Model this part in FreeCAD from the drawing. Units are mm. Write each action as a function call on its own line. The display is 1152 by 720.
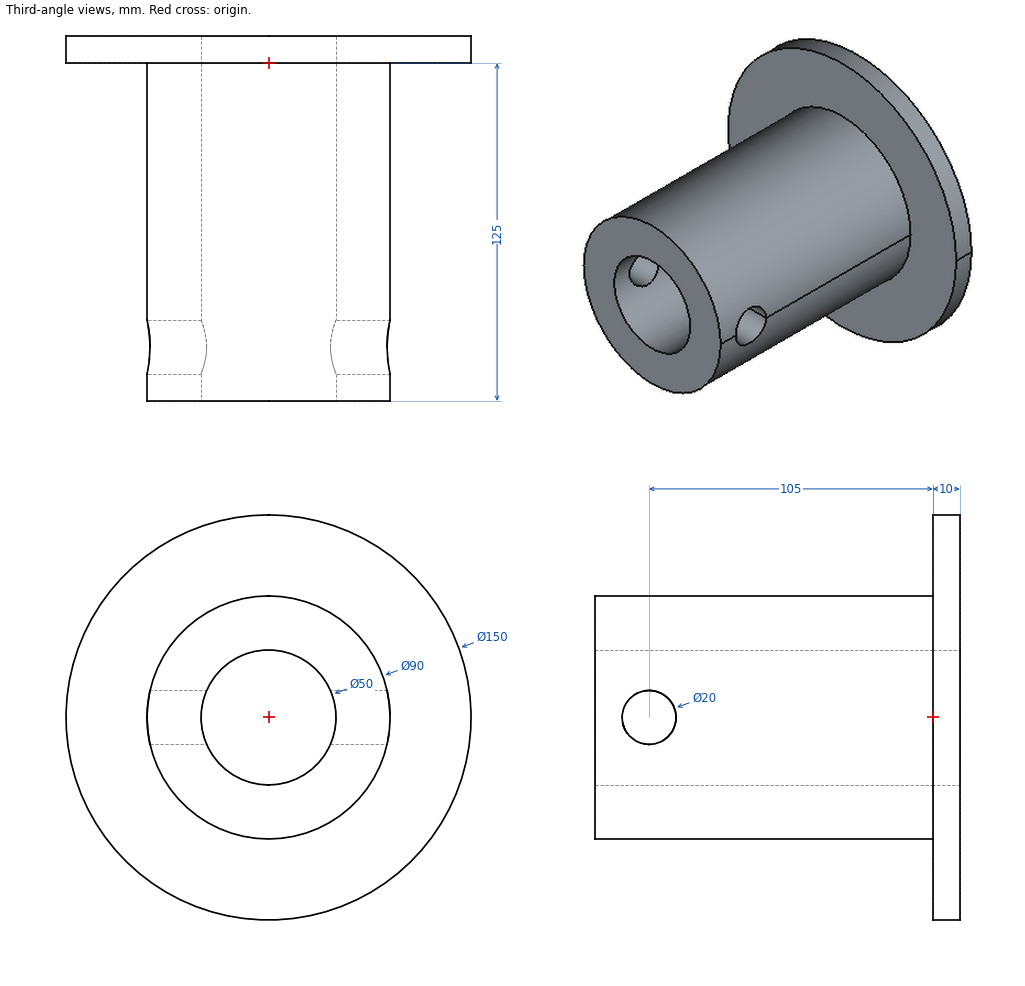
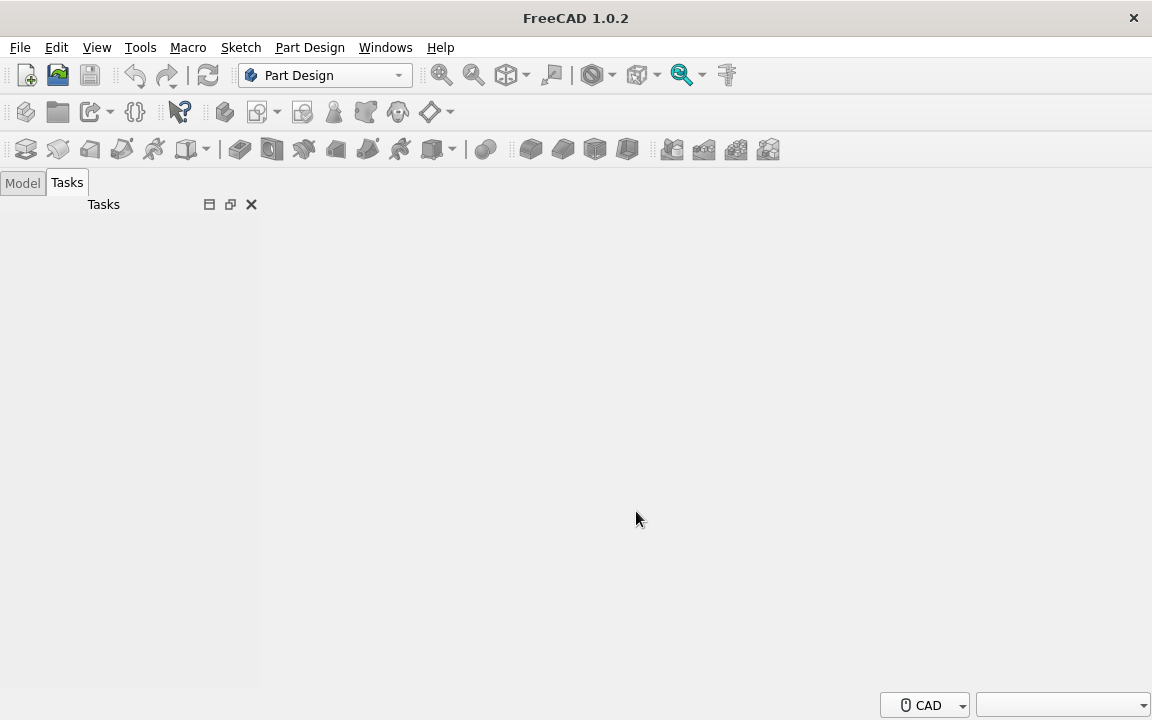
click(26, 76)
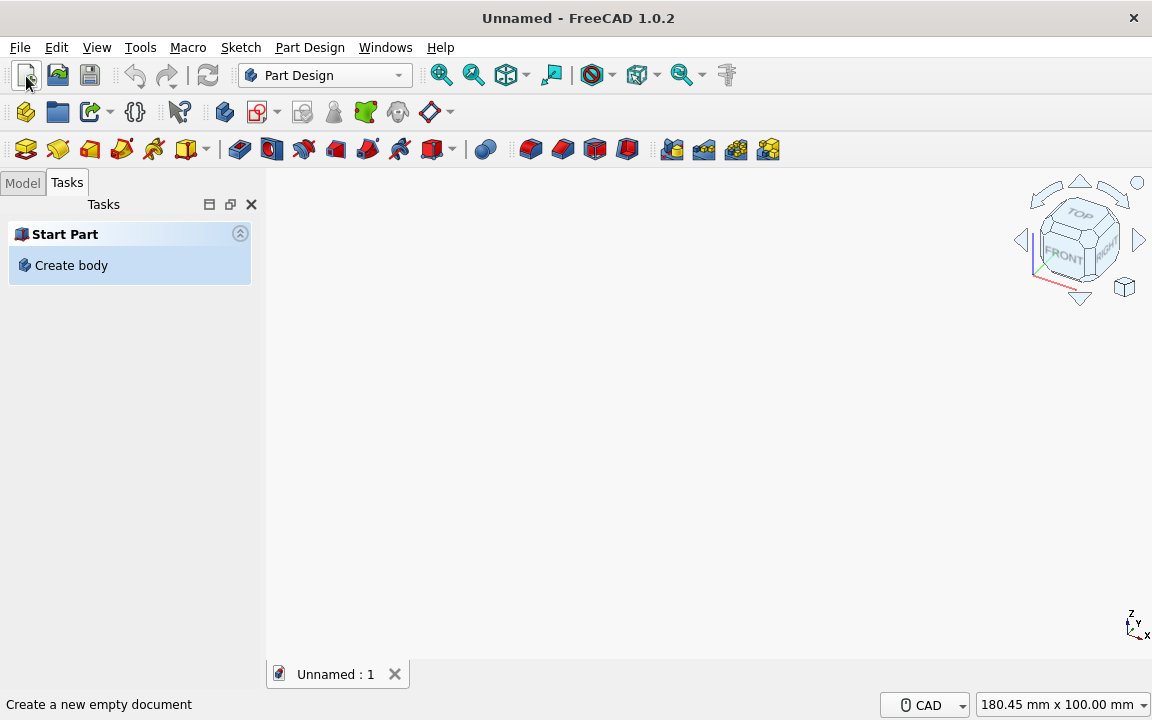
click(258, 112)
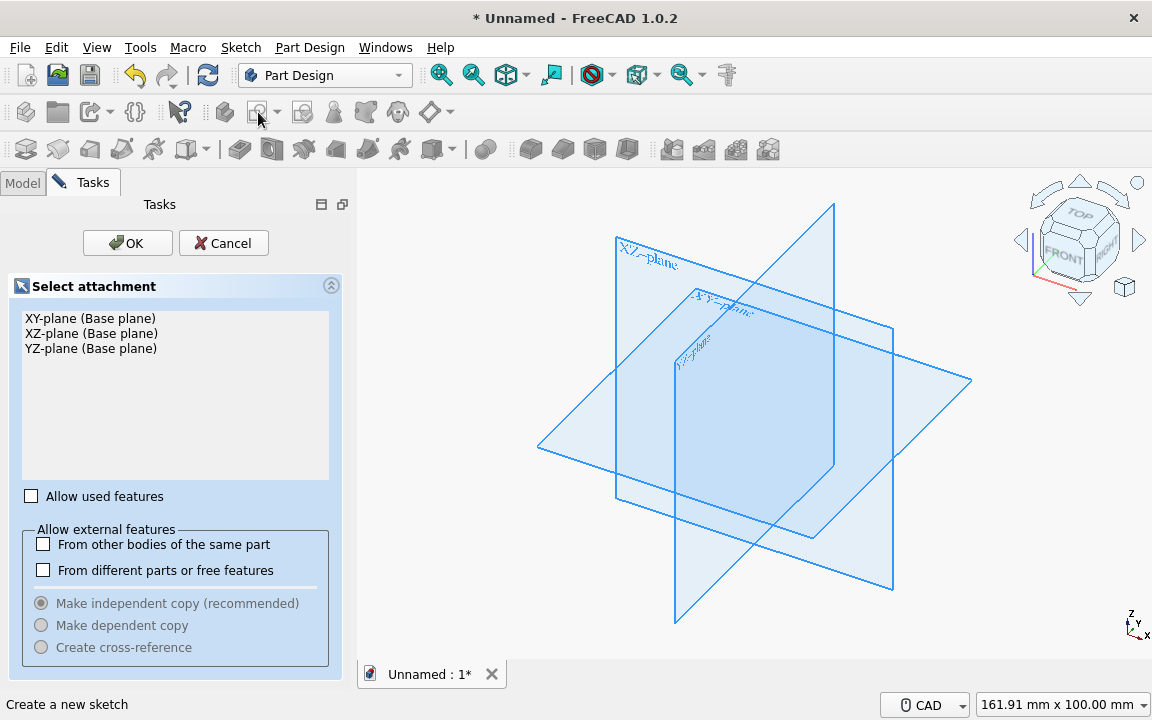
click(82, 334)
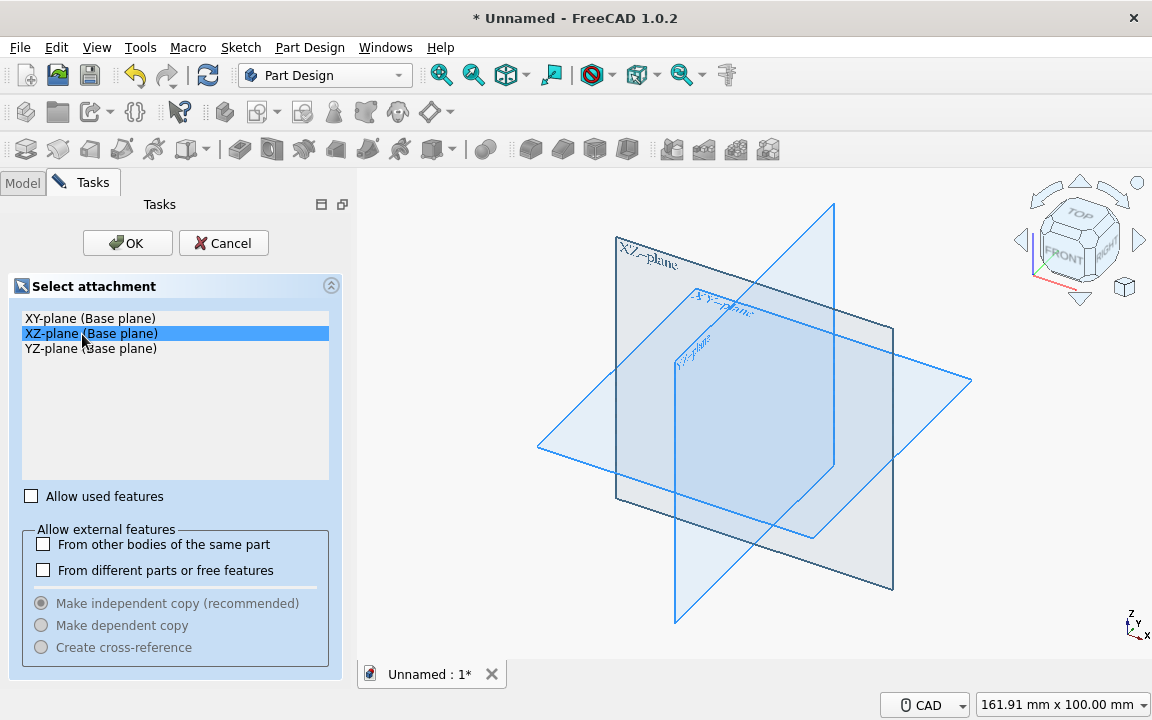
click(128, 243)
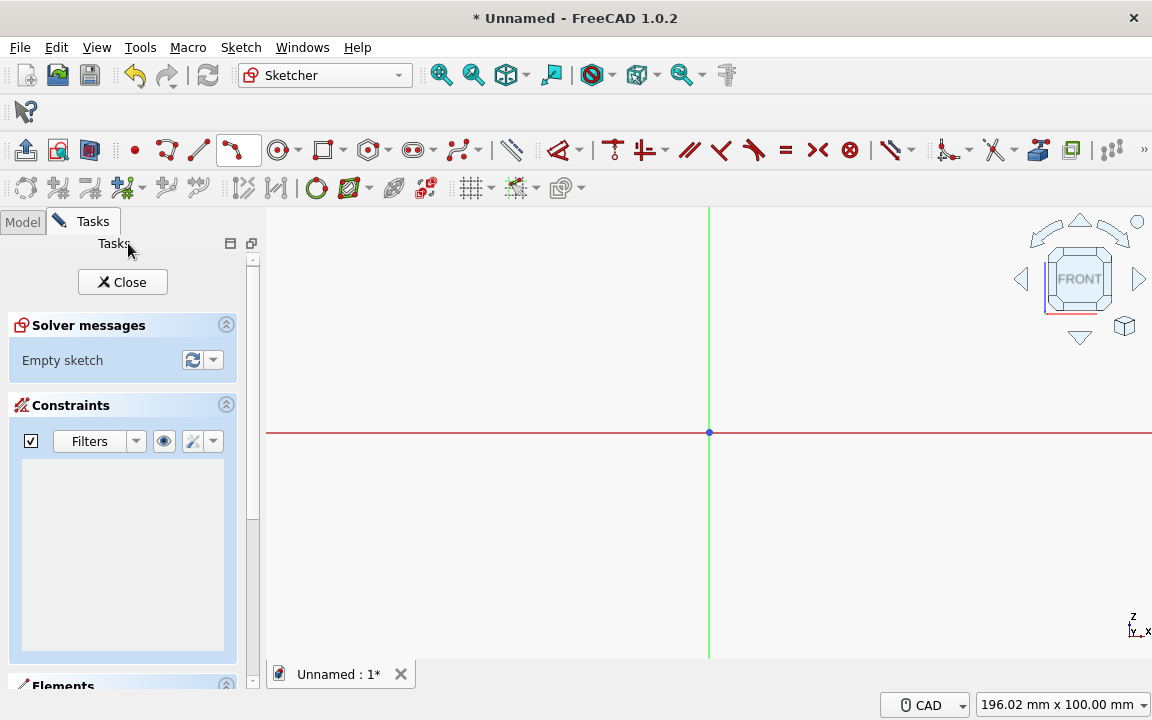
scroll(585, 433, down, 4)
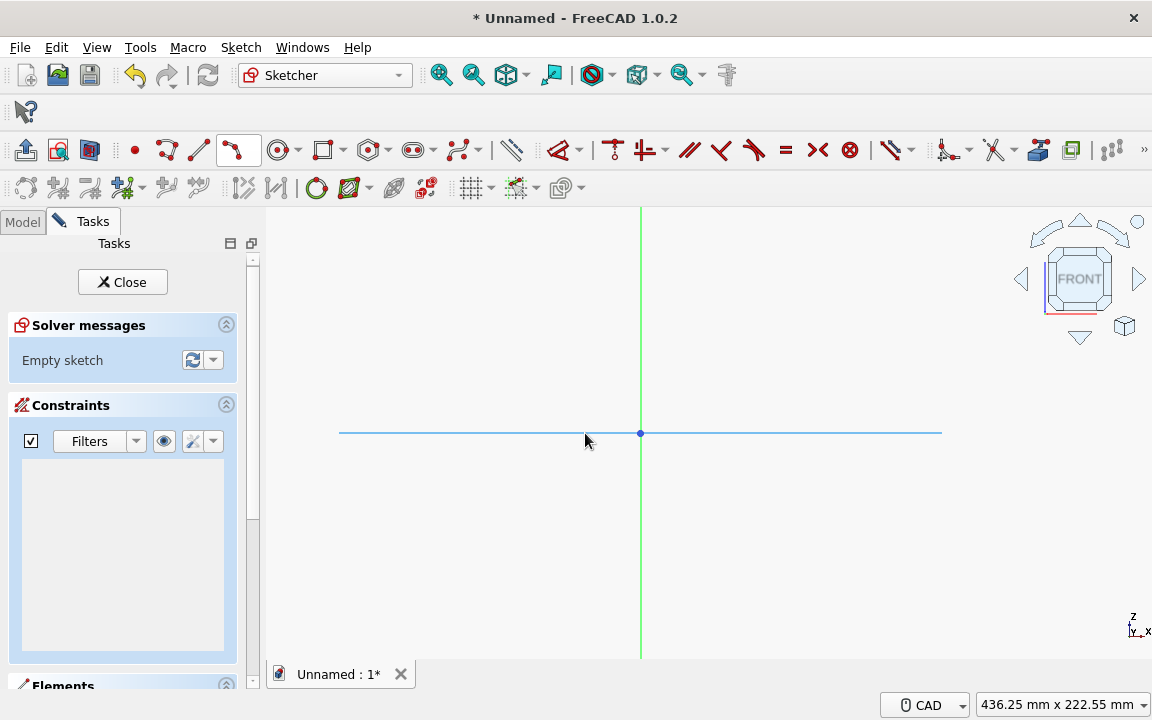
click(278, 150)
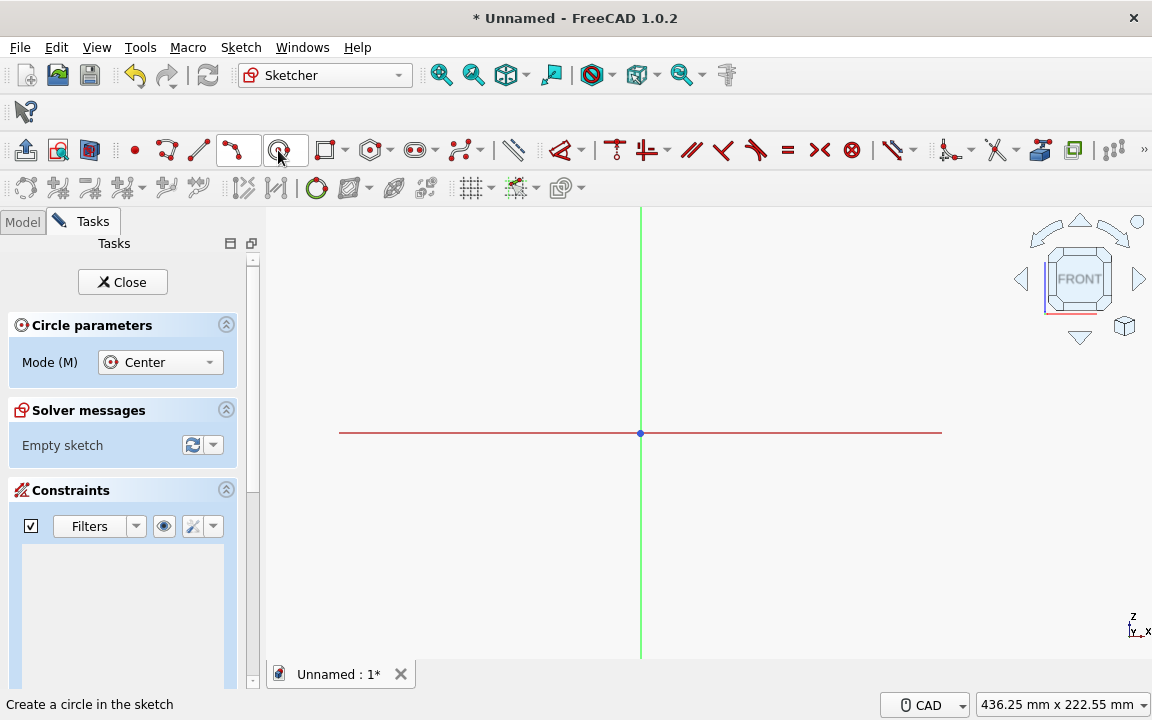
click(641, 433)
click(749, 326)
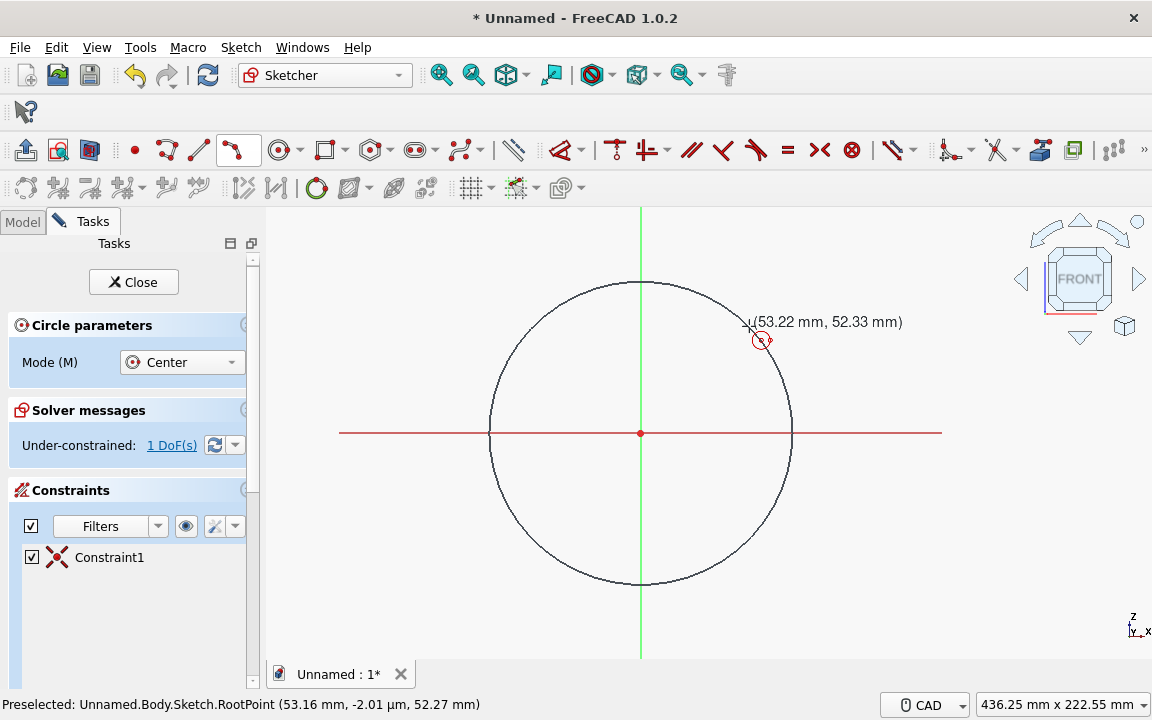
click(641, 433)
click(677, 397)
key(Escape)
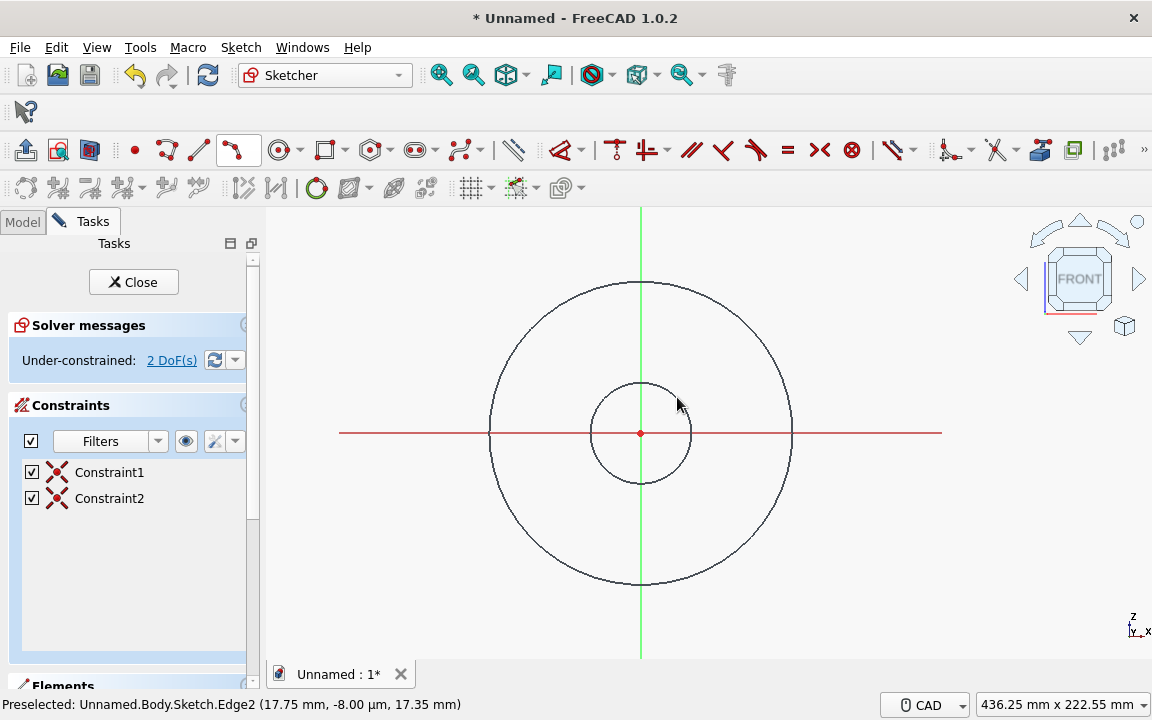
click(560, 150)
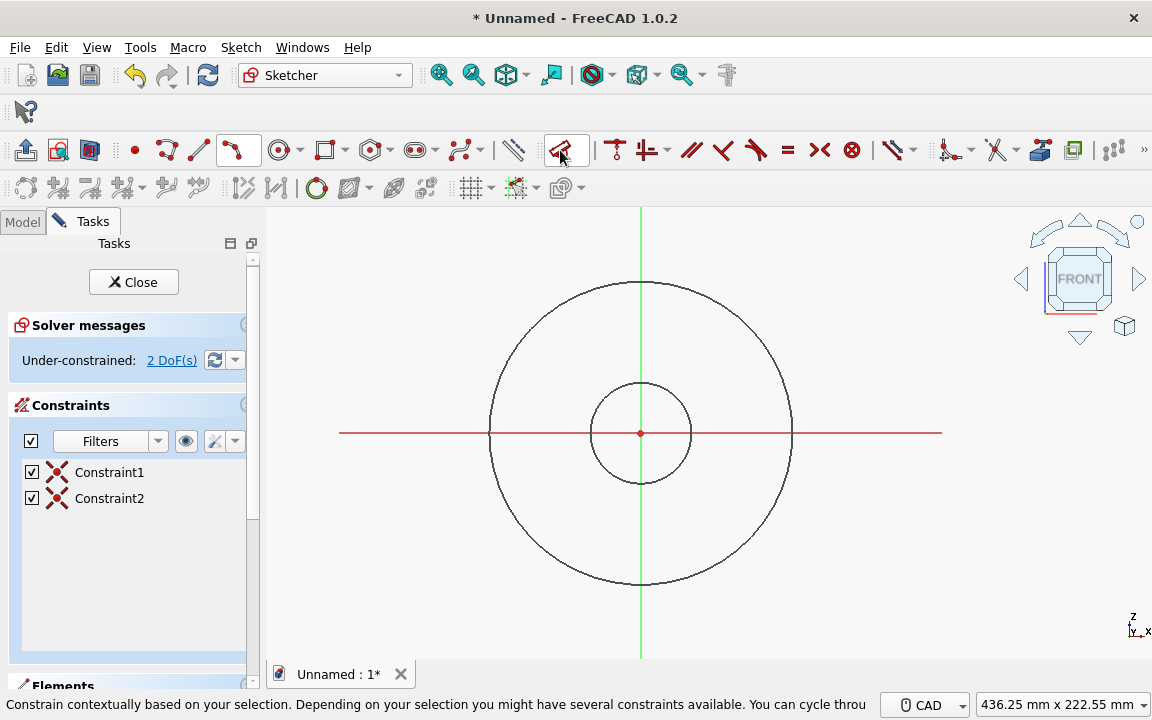
click(748, 326)
click(771, 303)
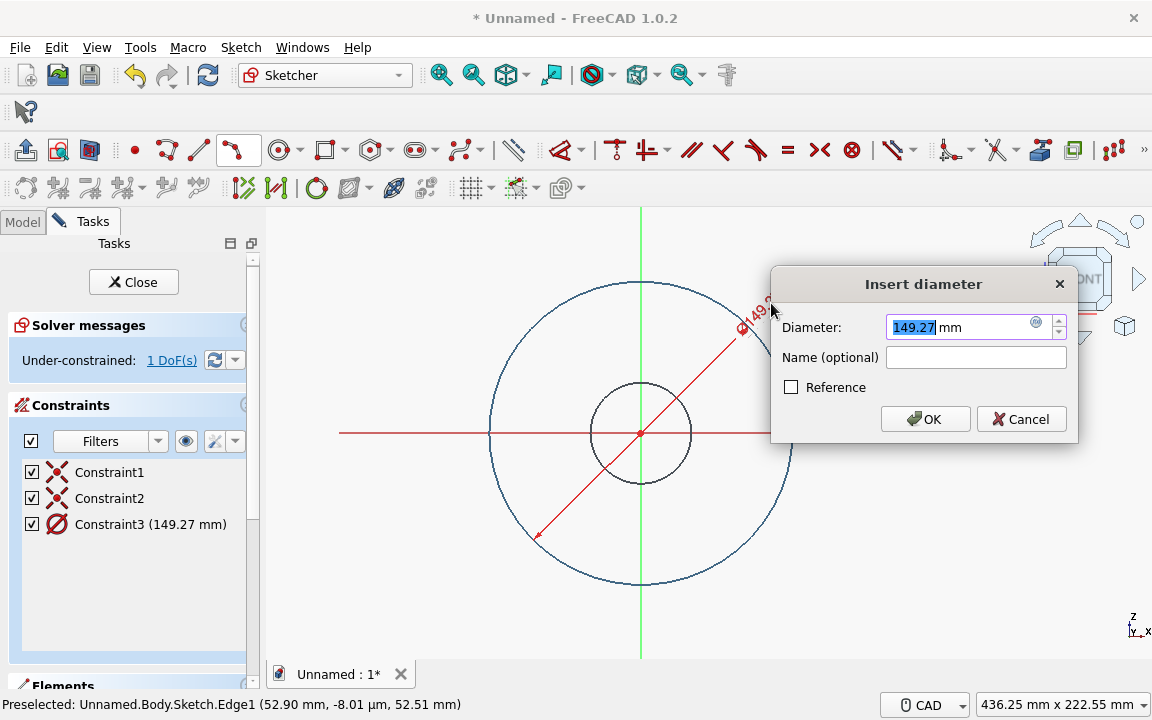
text(150)
key(Return)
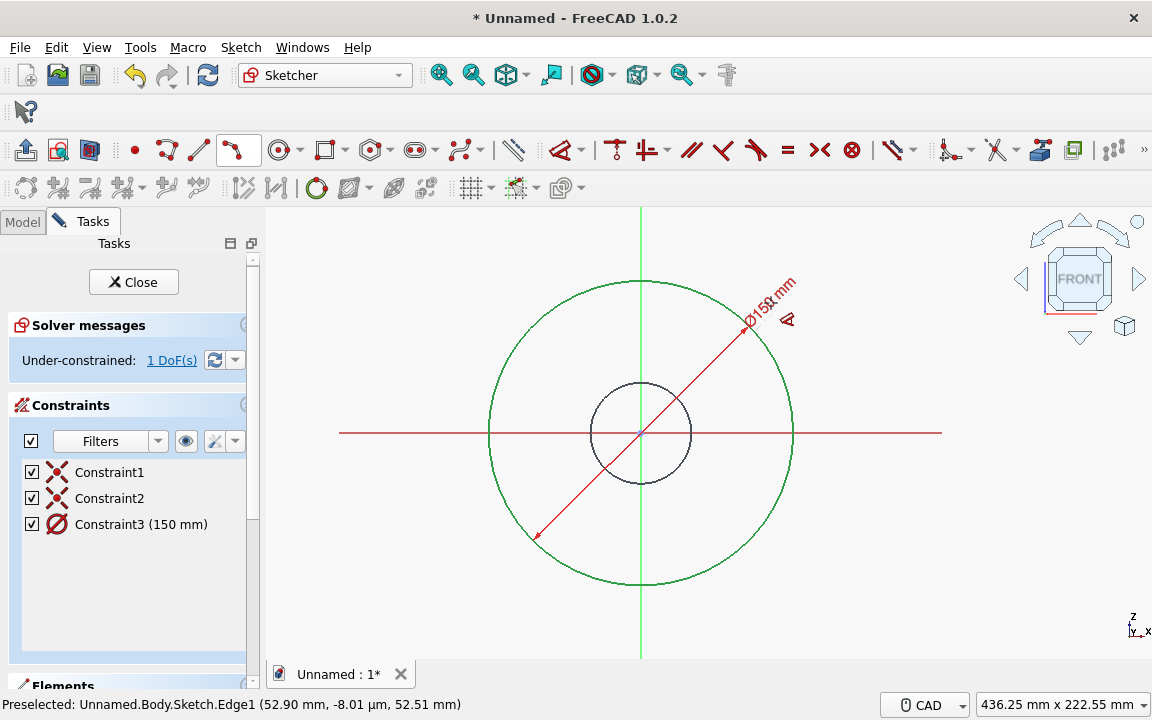
click(676, 397)
click(698, 374)